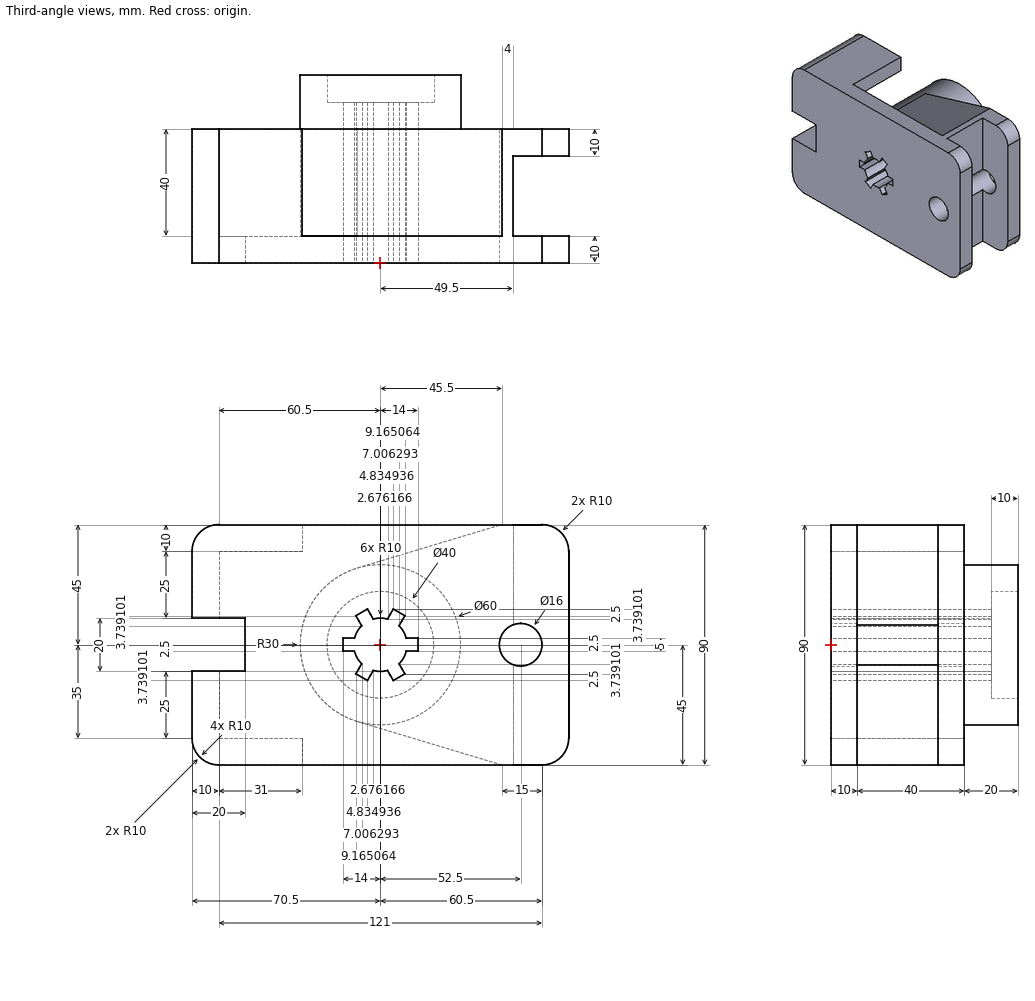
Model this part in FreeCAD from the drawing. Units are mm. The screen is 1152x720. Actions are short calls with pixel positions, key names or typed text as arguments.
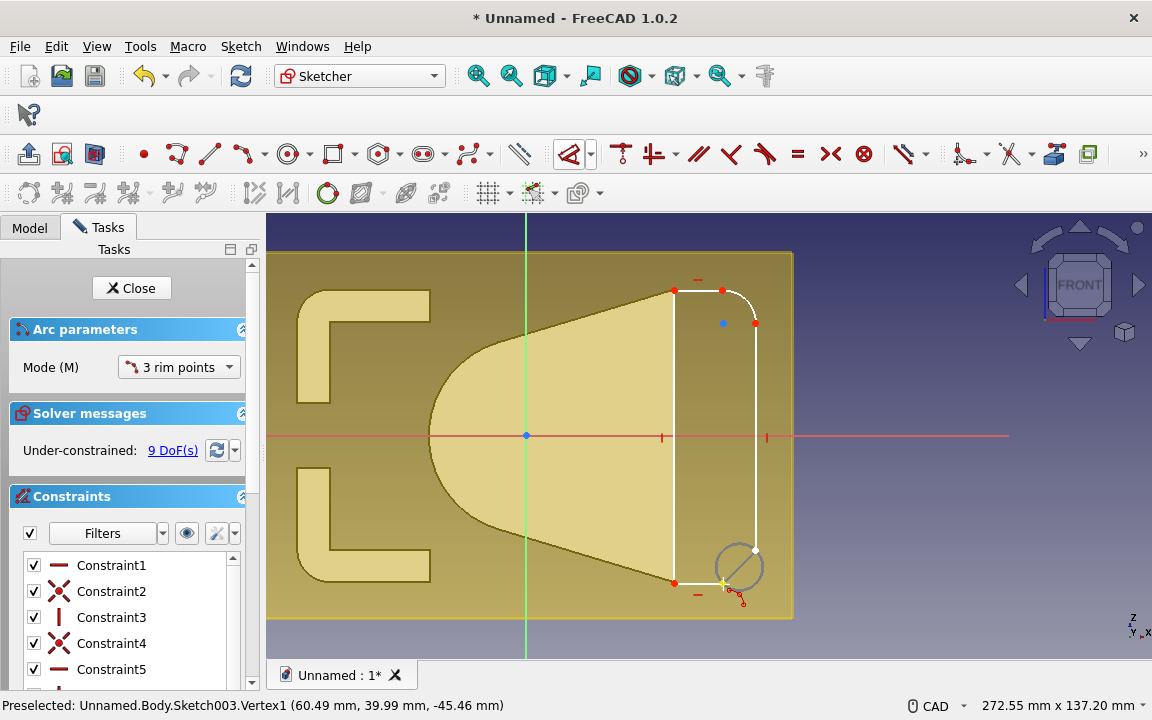
scroll(746, 573, up, 3)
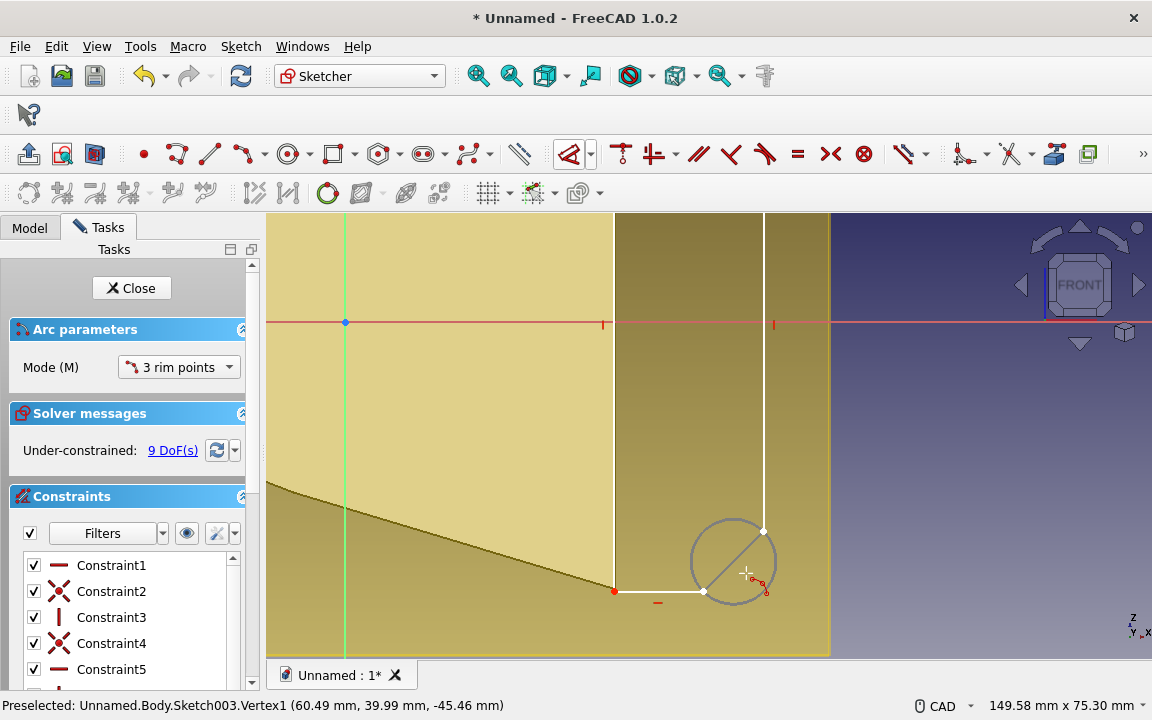
click(745, 572)
key(Escape)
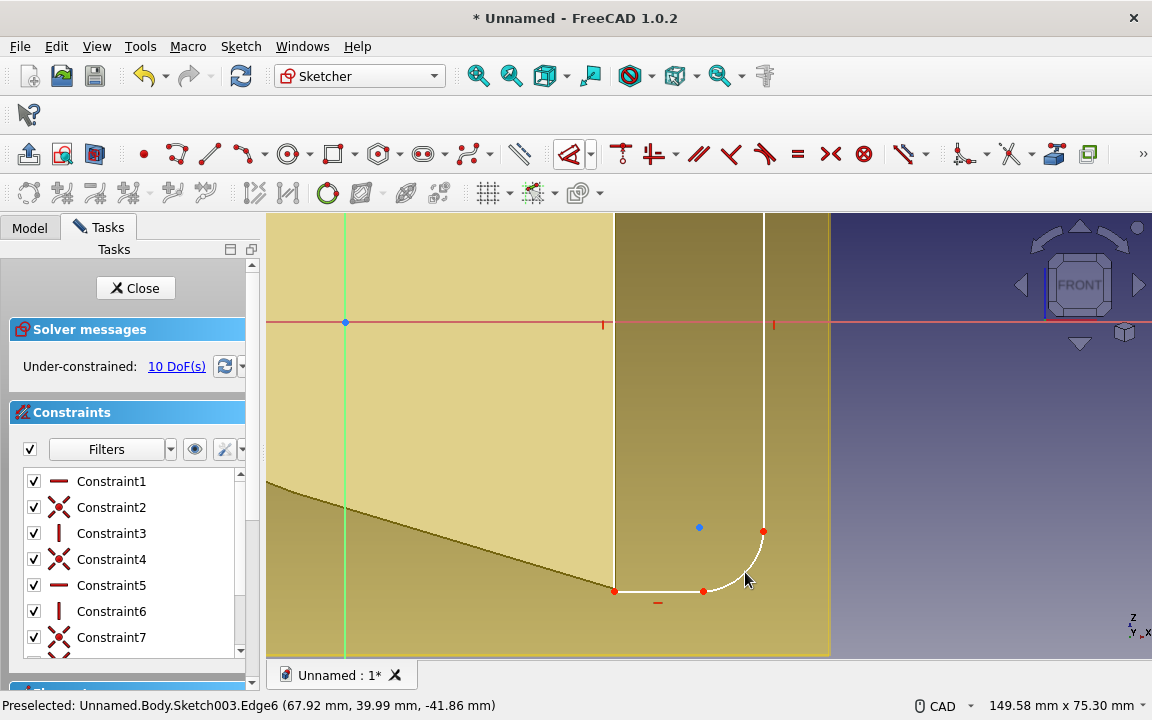
click(677, 592)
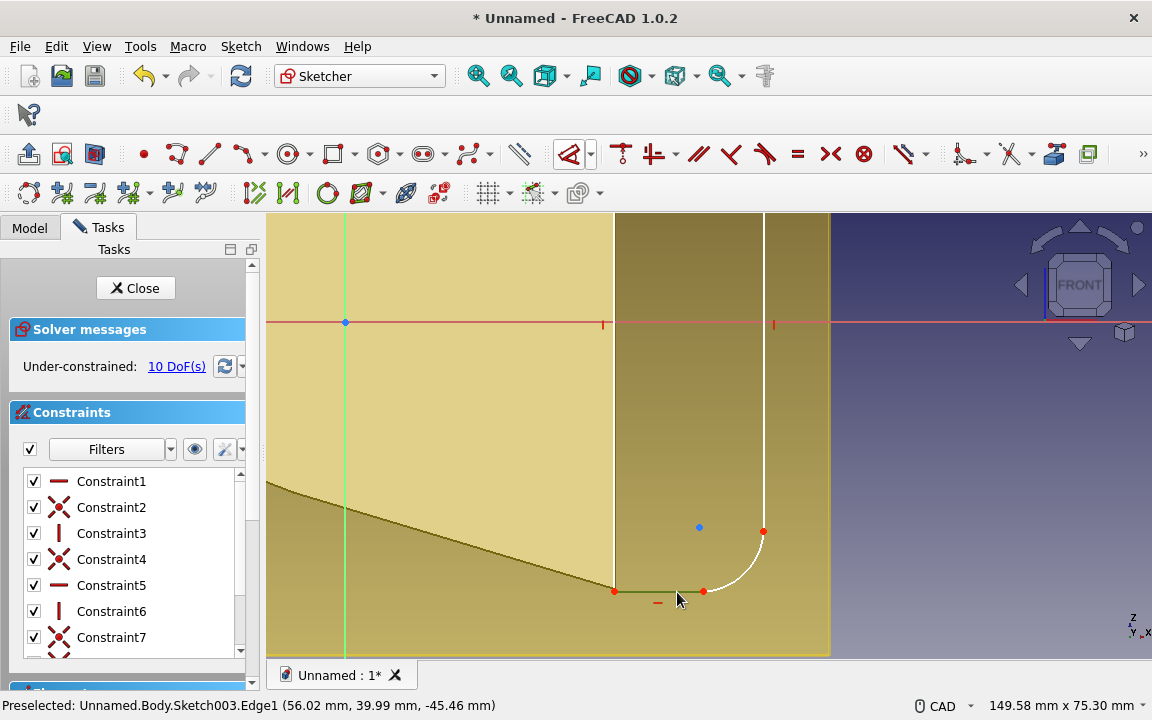
click(730, 584)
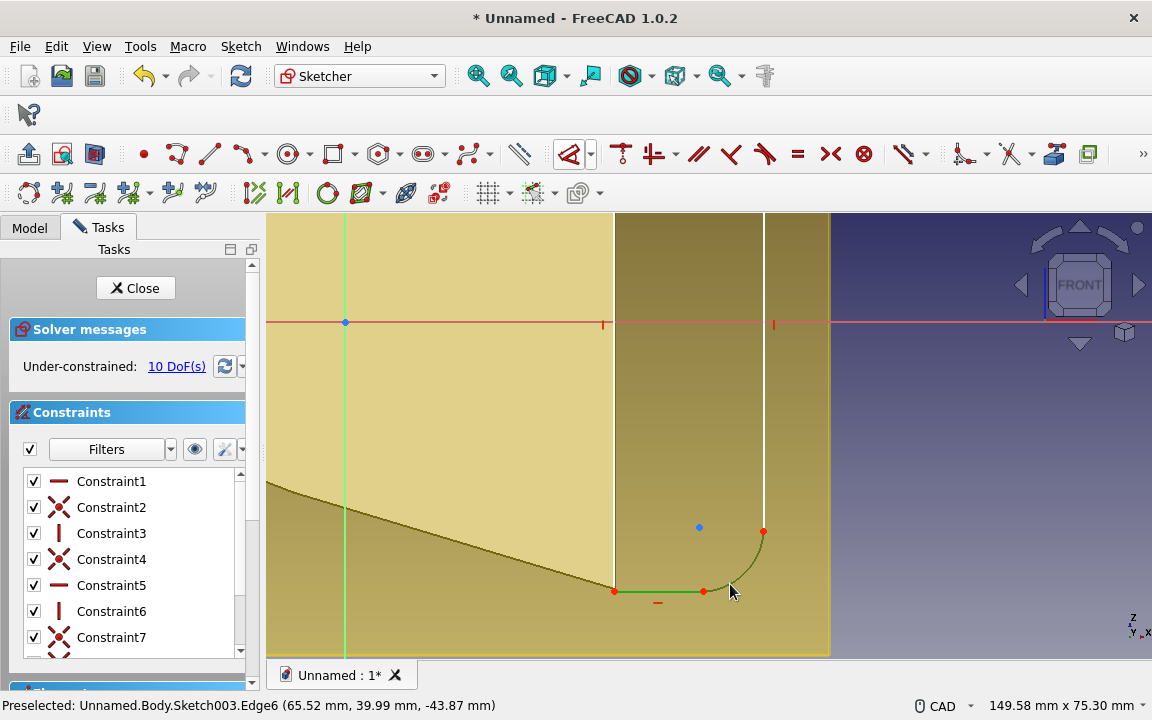
click(765, 154)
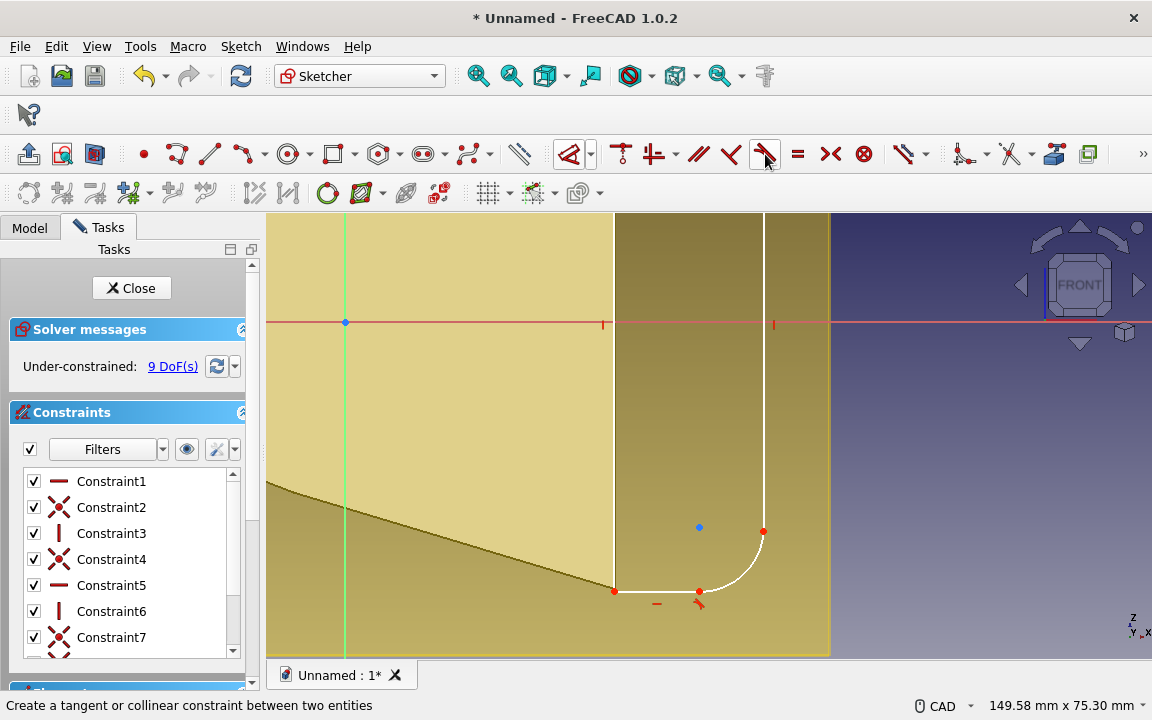
scroll(746, 574, down, 3)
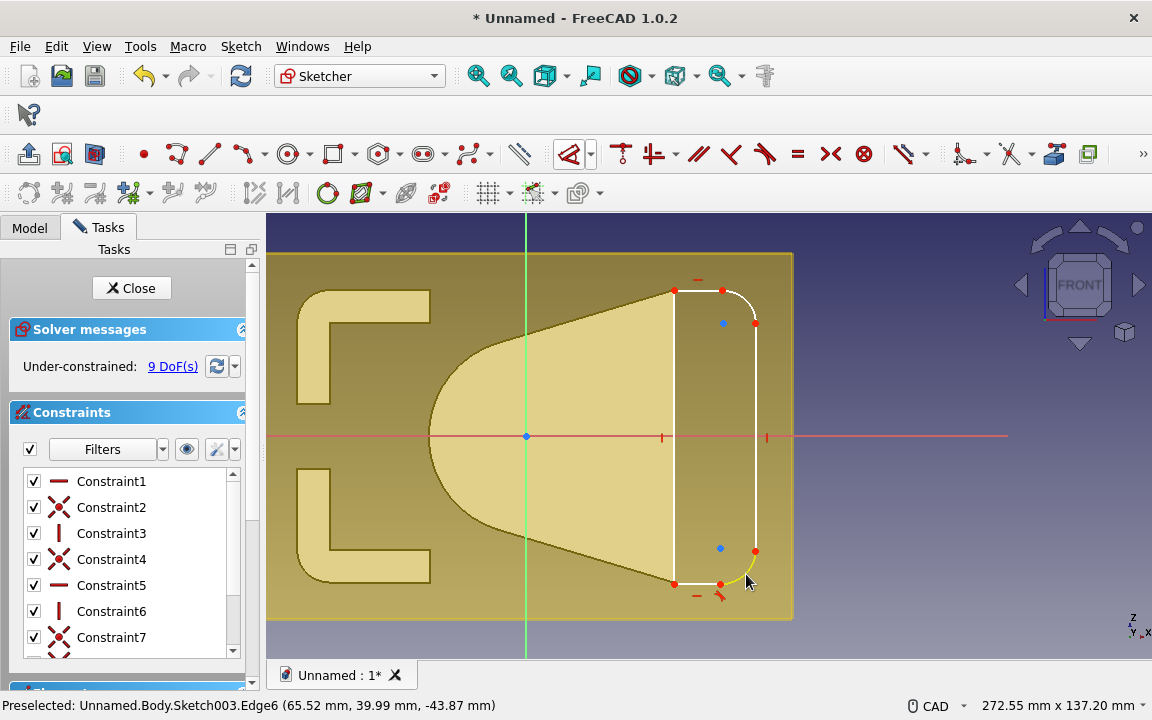
click(689, 291)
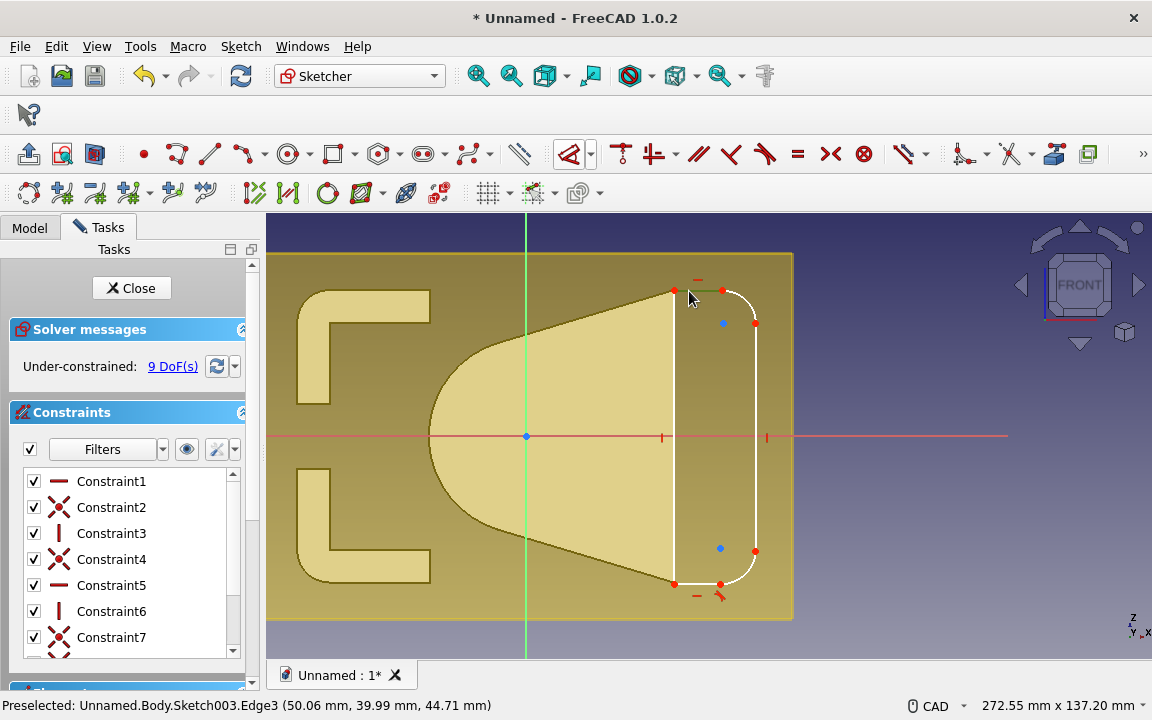
click(752, 309)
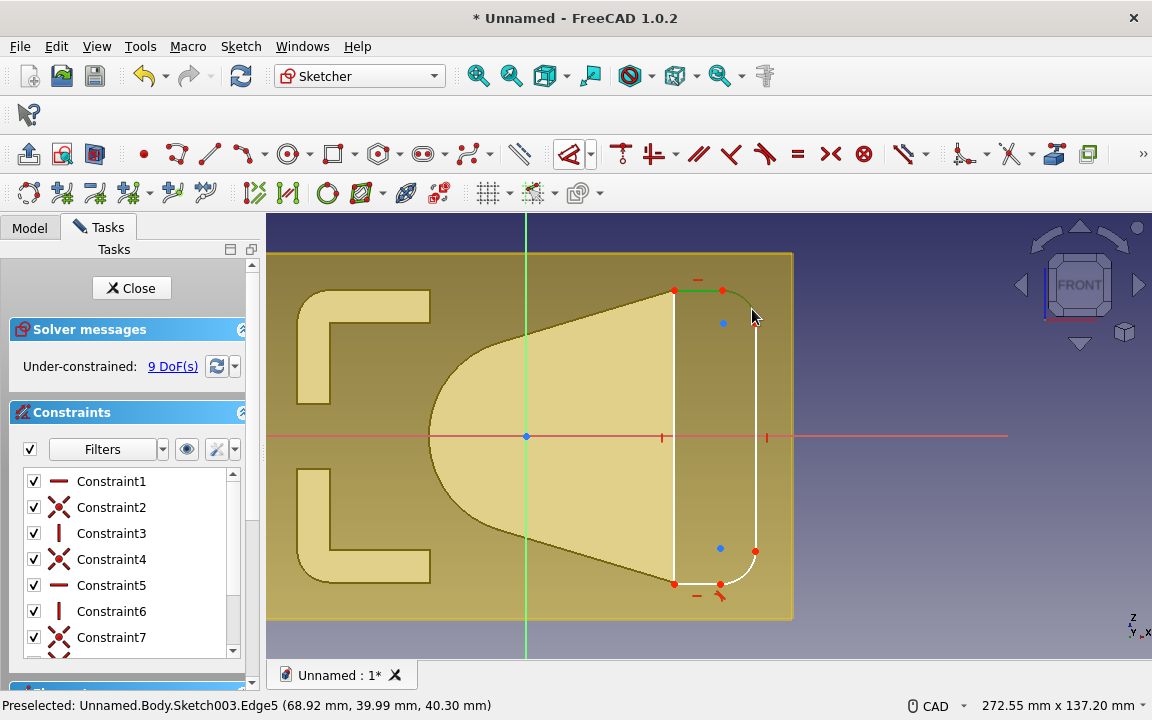
click(765, 154)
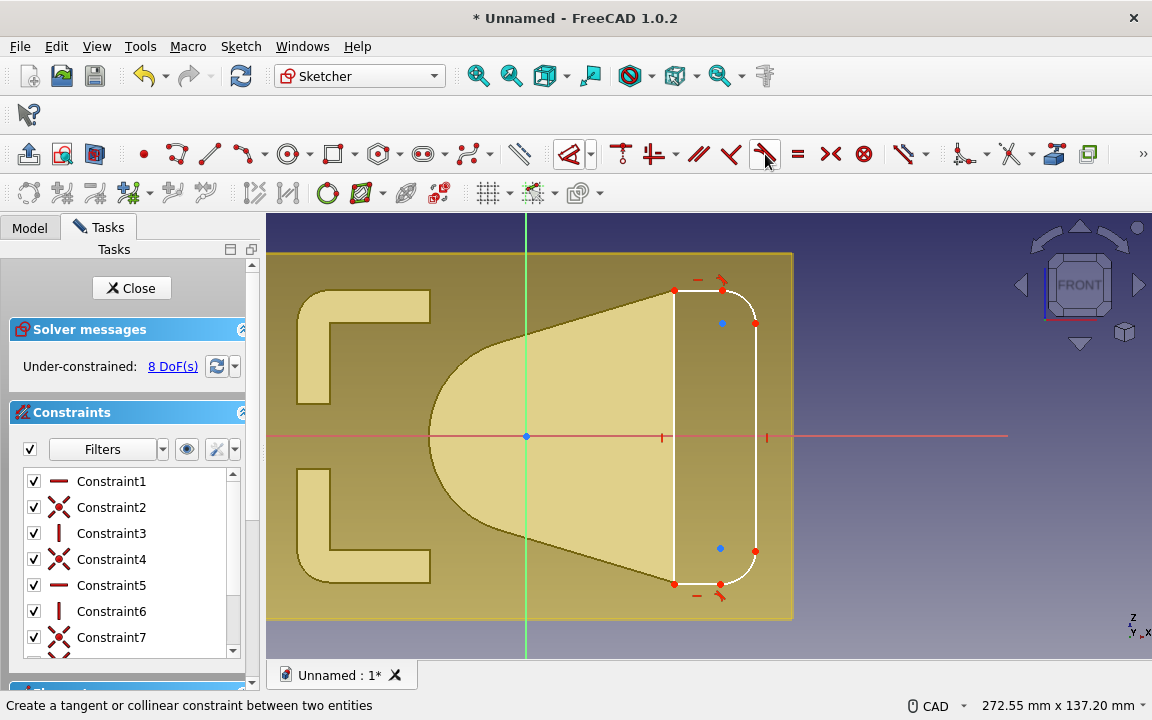
click(756, 392)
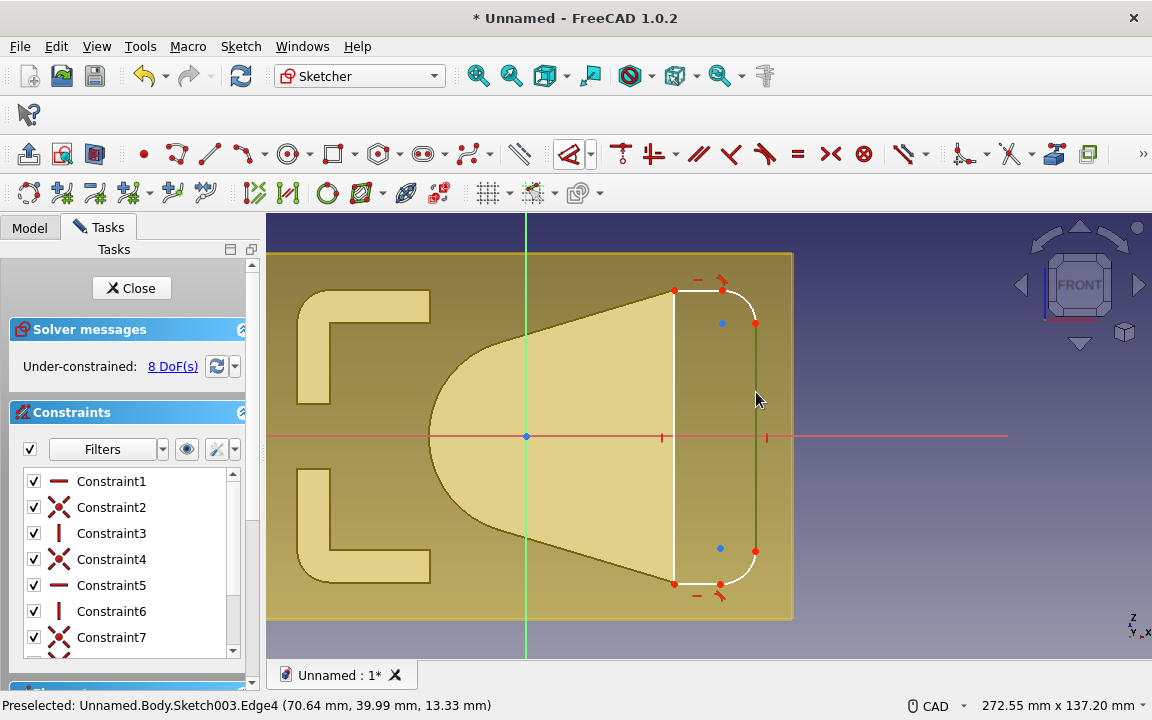
click(752, 309)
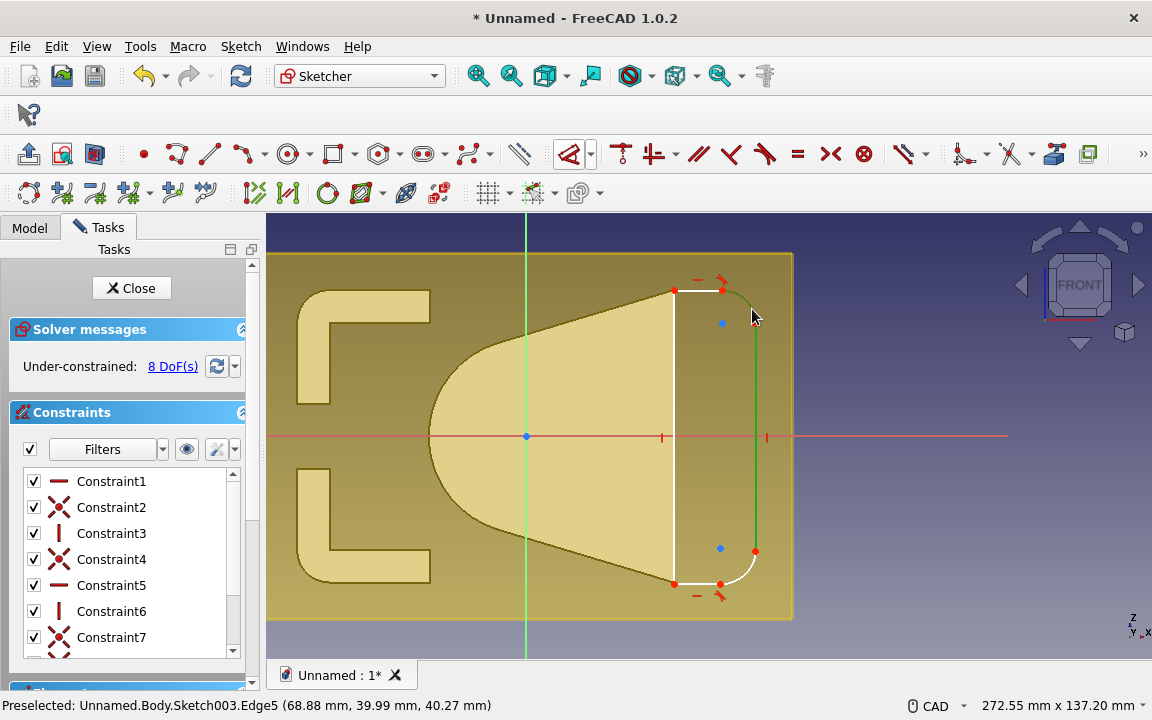
click(765, 154)